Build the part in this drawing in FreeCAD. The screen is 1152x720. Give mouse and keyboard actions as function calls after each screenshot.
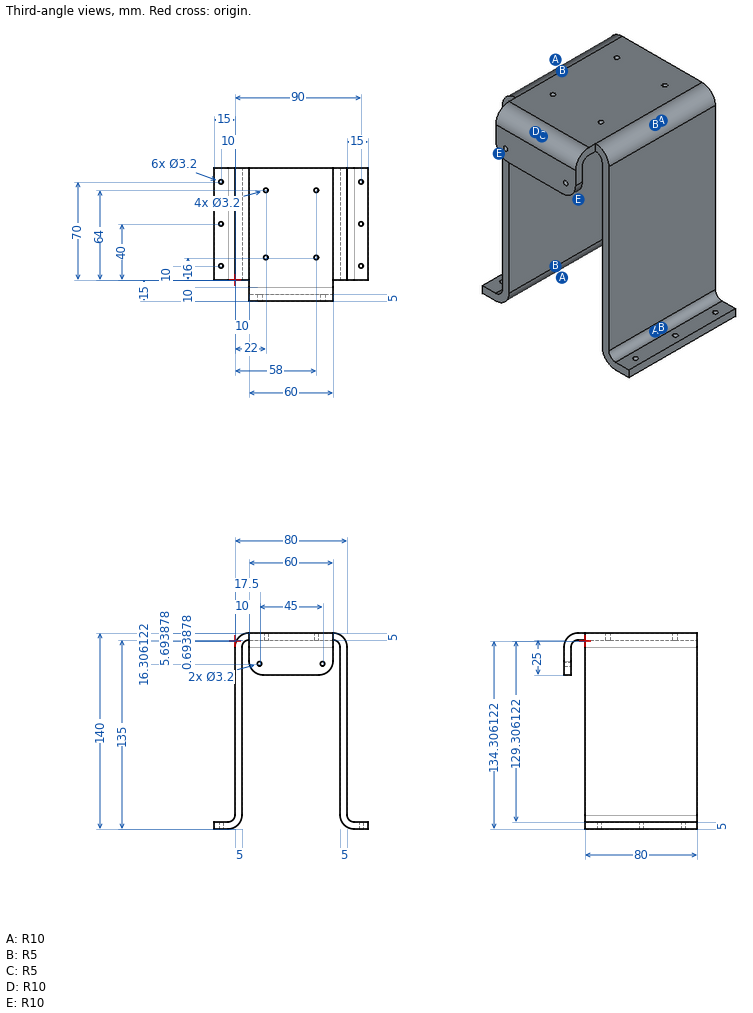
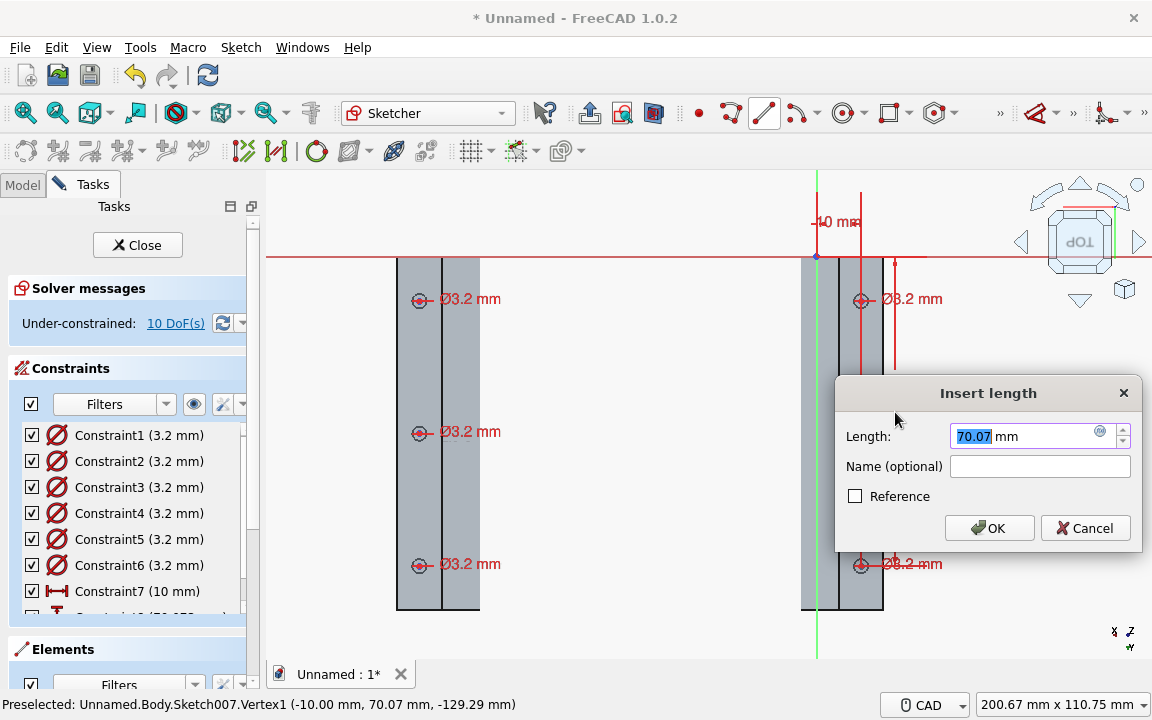
text(70)
key(Return)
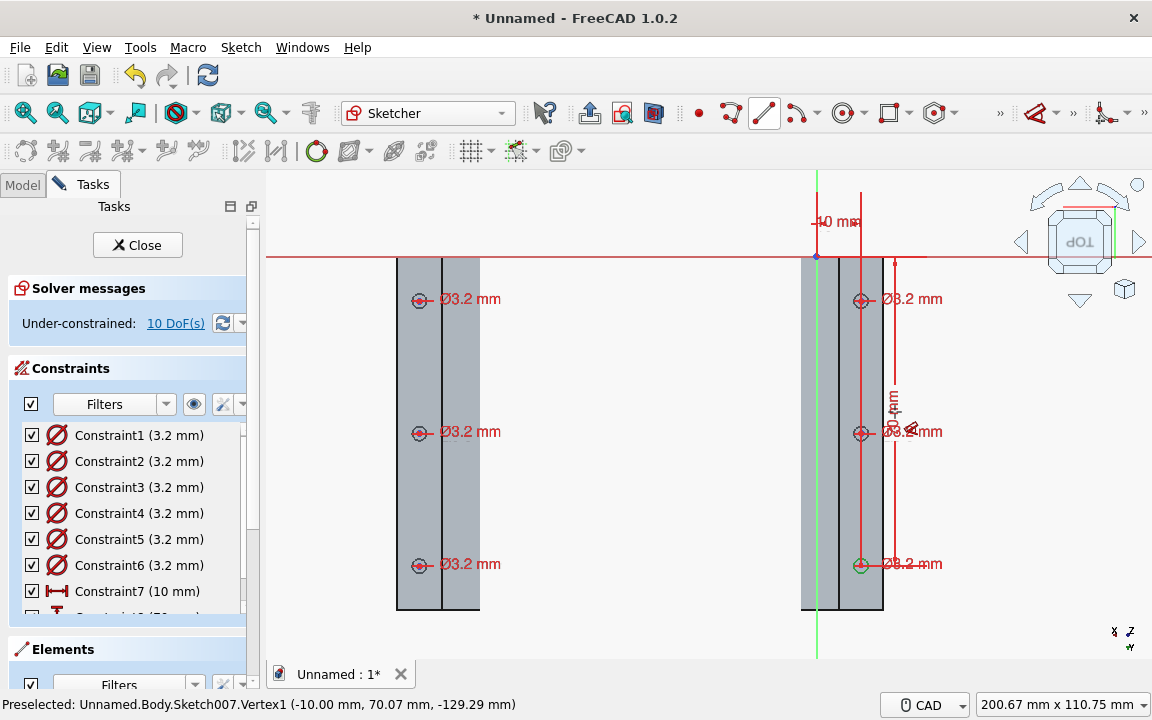
click(861, 434)
click(839, 468)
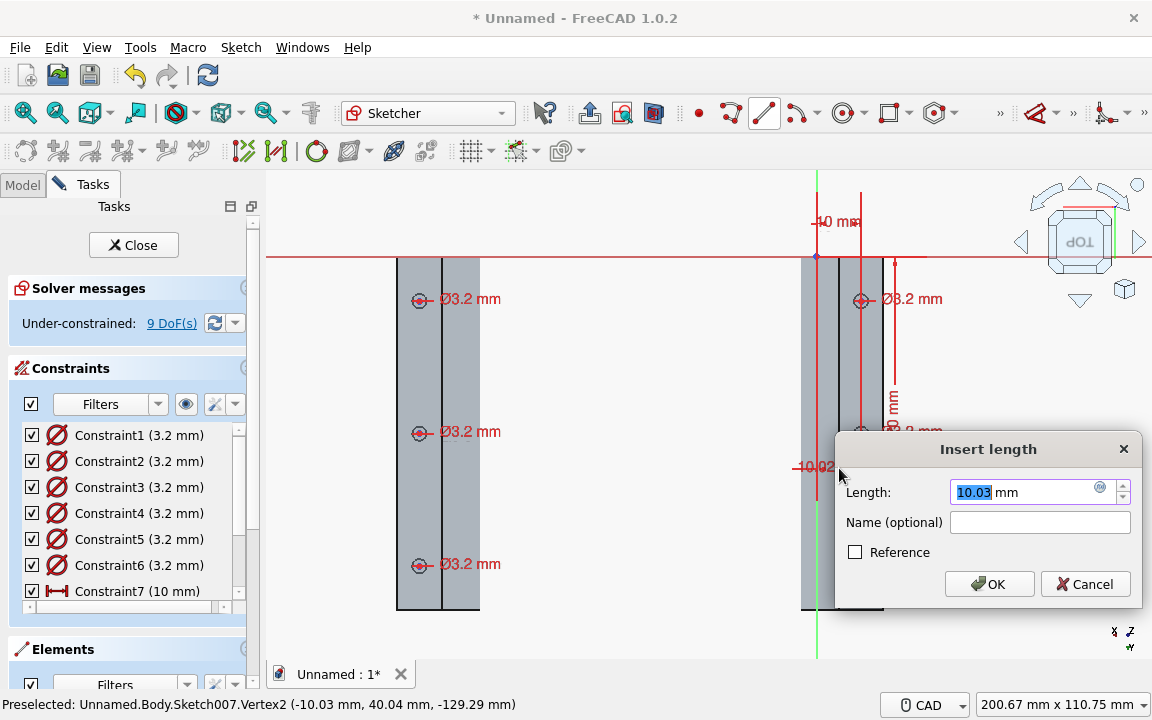
text(10)
key(Return)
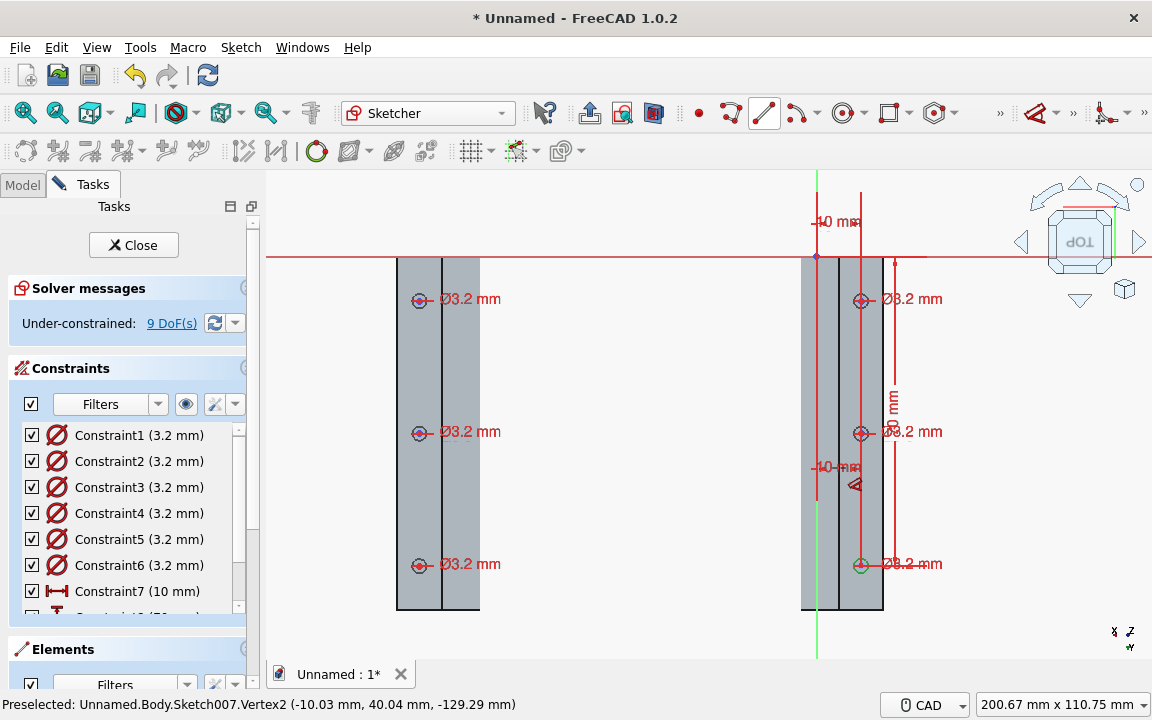
click(861, 434)
click(895, 345)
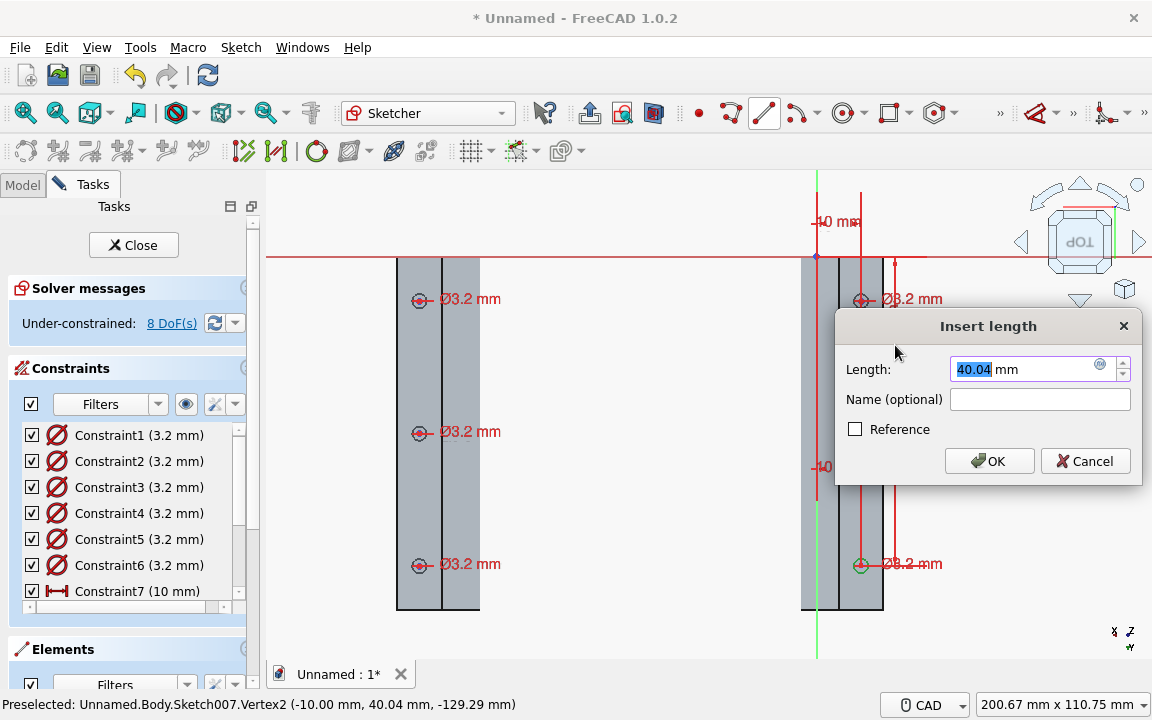
text(40)
key(Return)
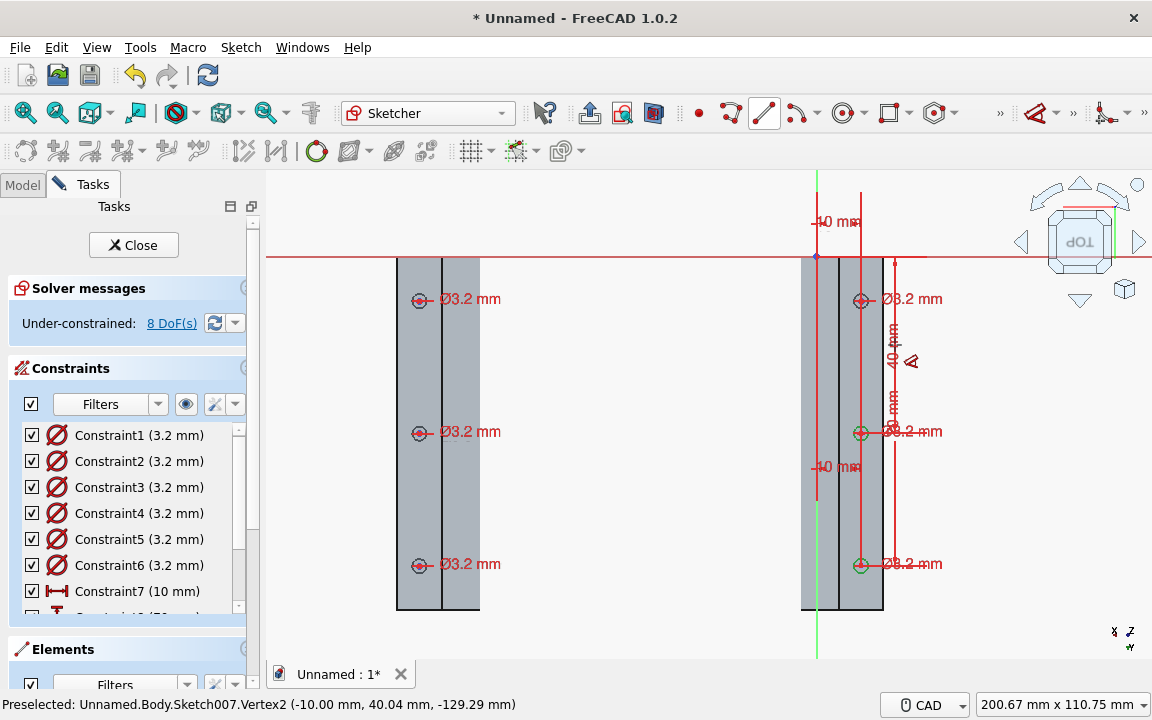
click(861, 301)
click(839, 199)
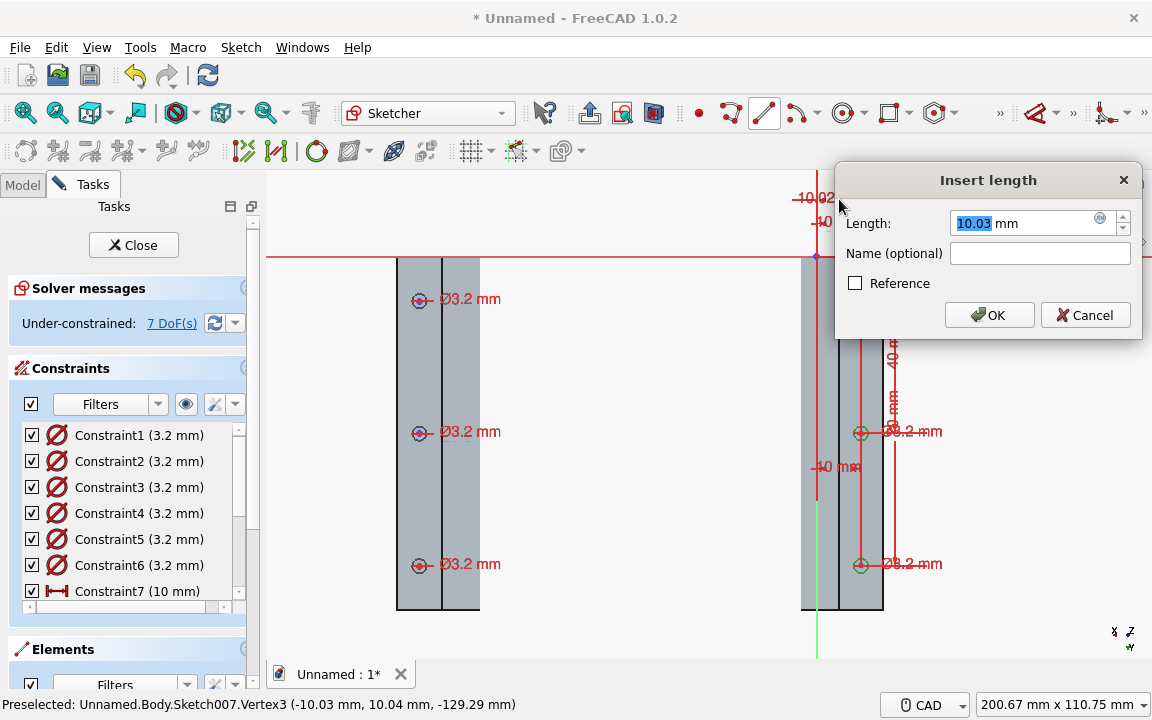
text(10)
key(Return)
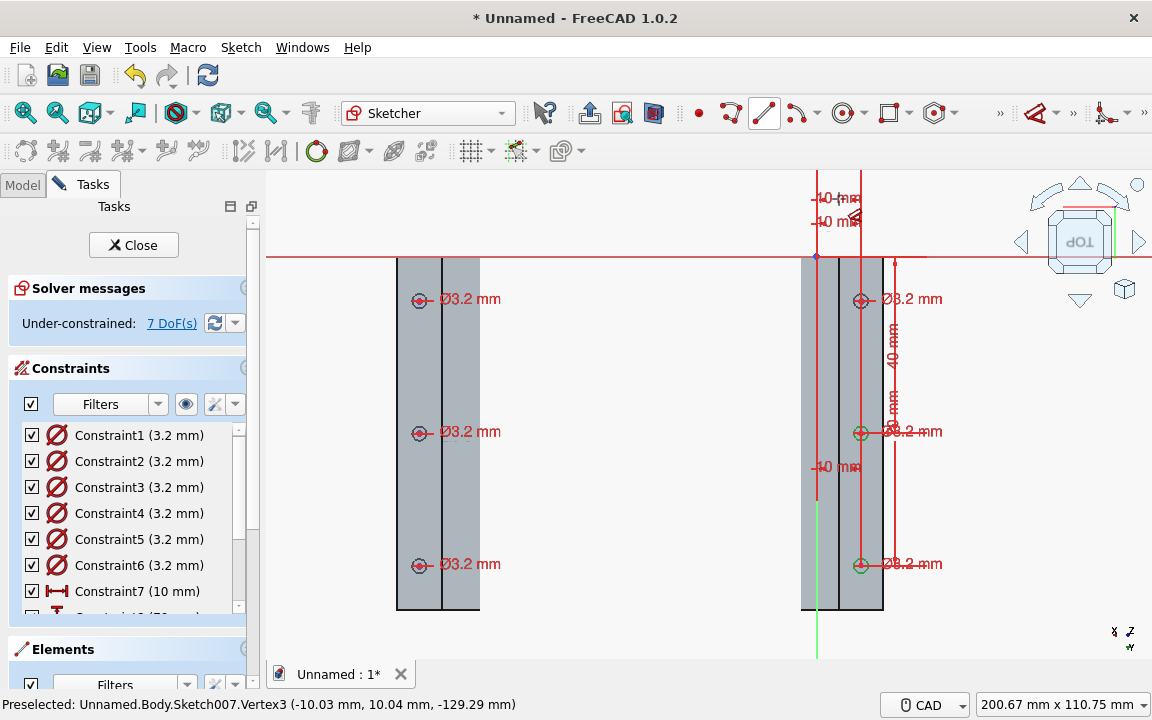
click(861, 301)
click(895, 279)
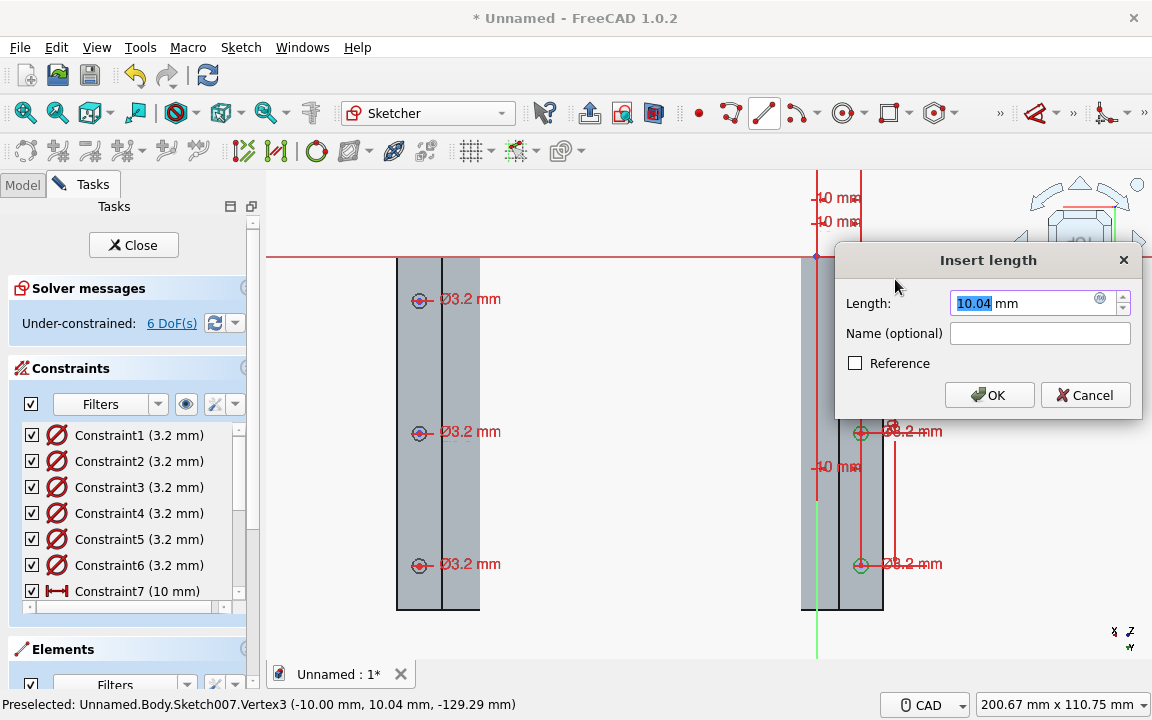
text(10)
key(Return)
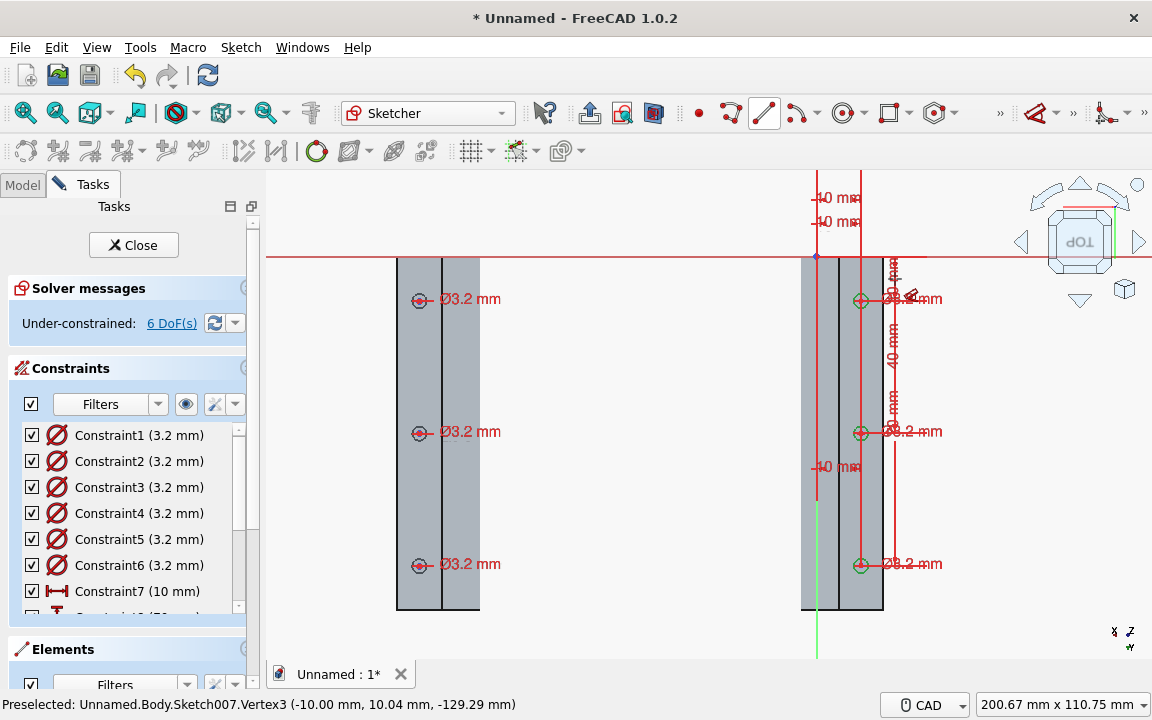
click(419, 566)
click(618, 223)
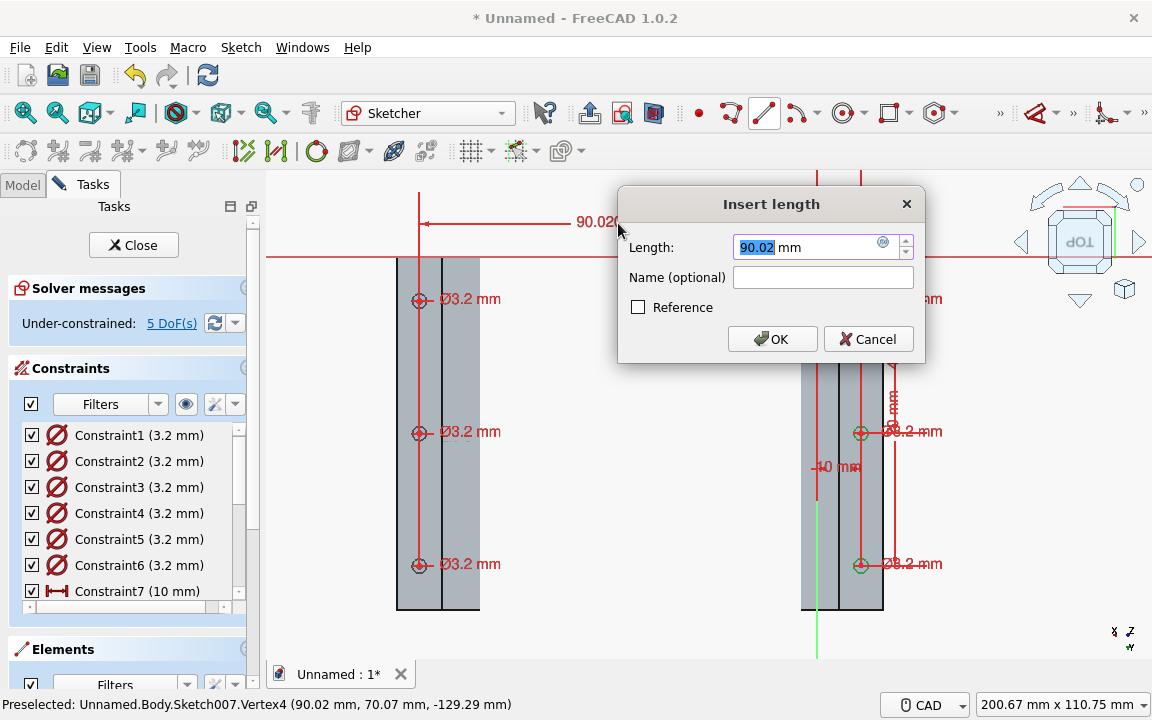
text(90)
key(Return)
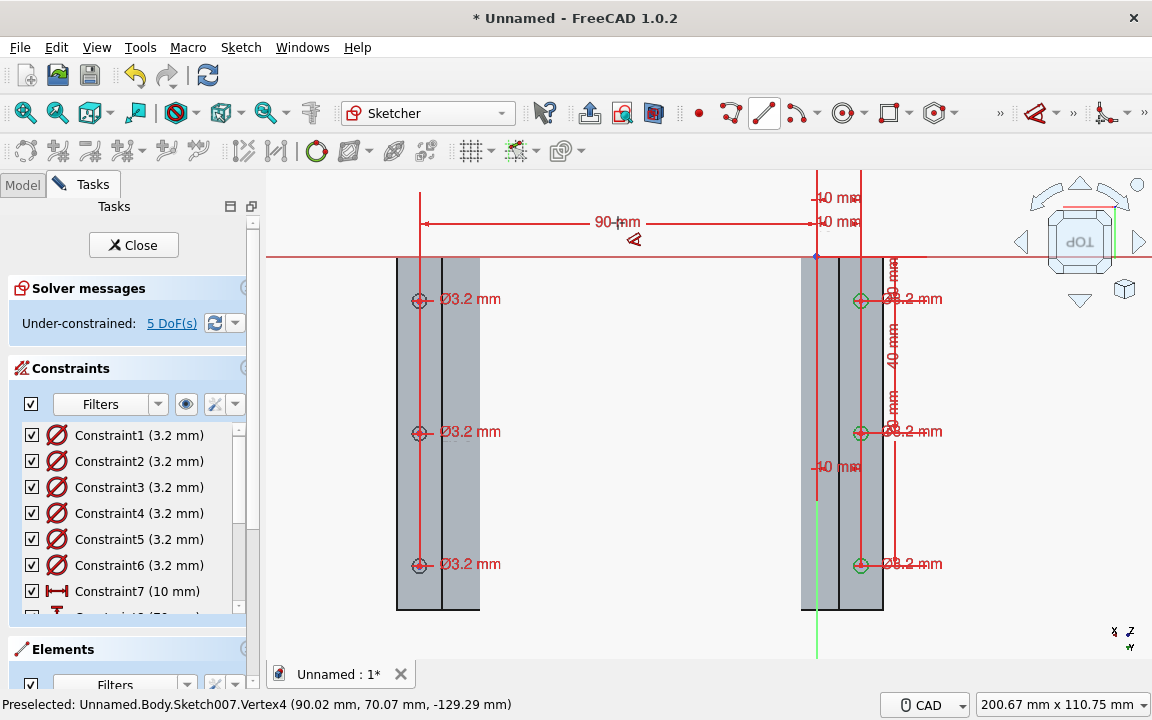
click(420, 566)
click(386, 412)